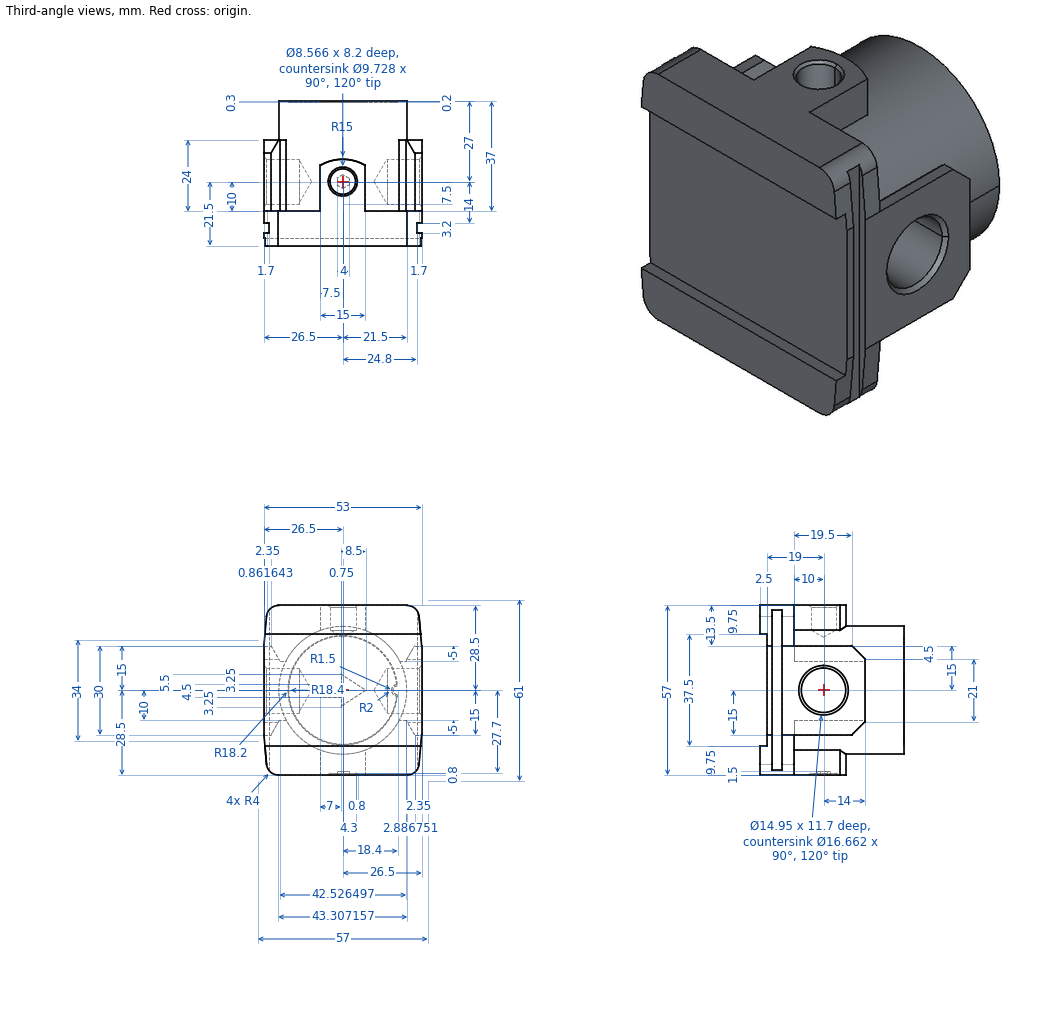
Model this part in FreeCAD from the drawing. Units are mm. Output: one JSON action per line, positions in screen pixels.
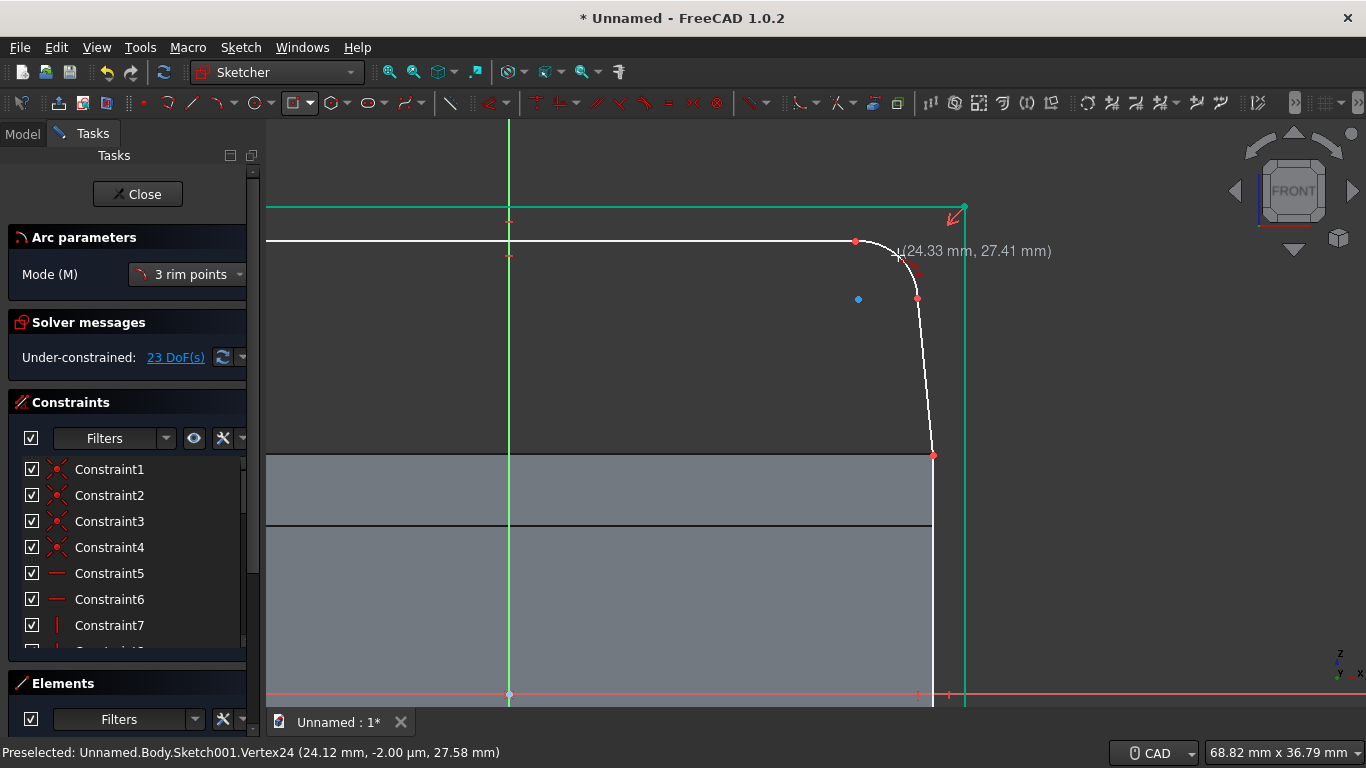
{"action": "scroll", "coordinate": [886, 249], "scroll_direction": "down", "scroll_amount": 5}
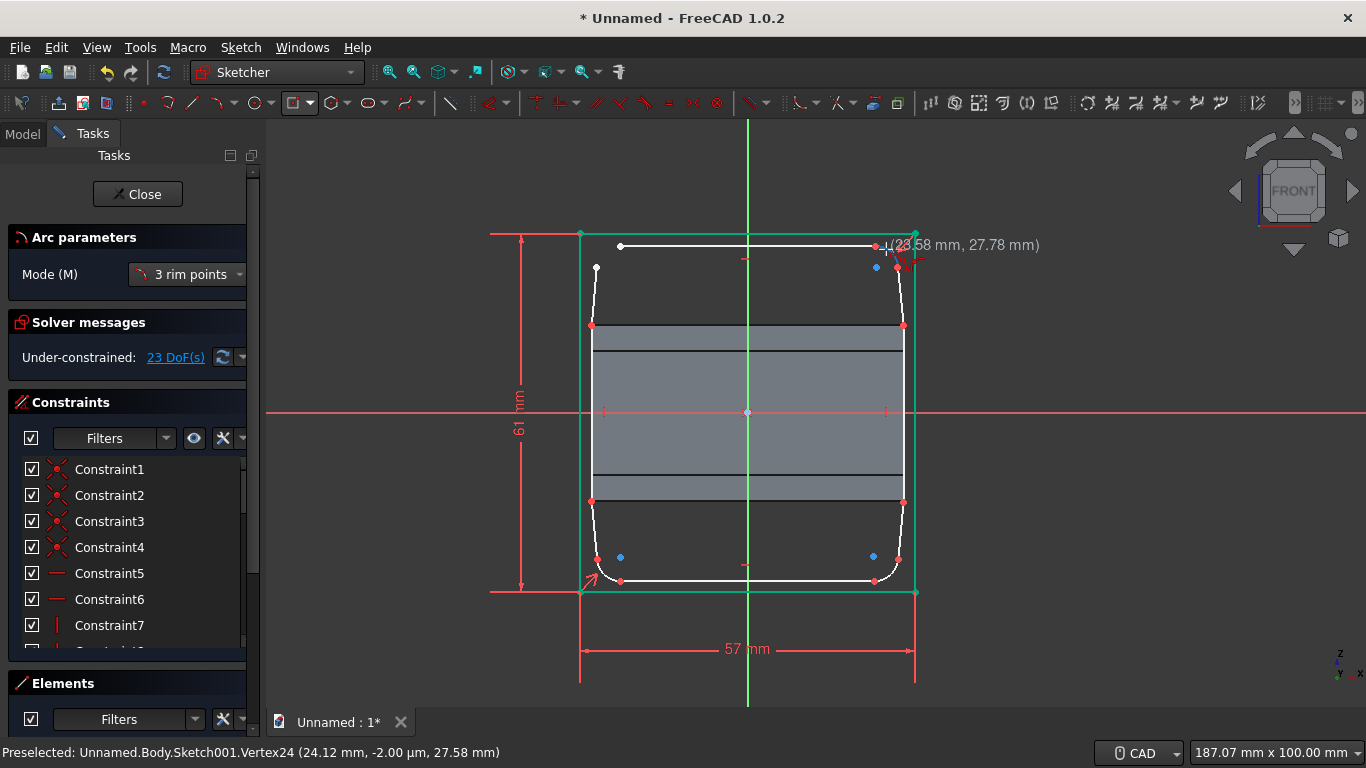
{"action": "scroll", "coordinate": [620, 245], "scroll_direction": "up", "scroll_amount": 2}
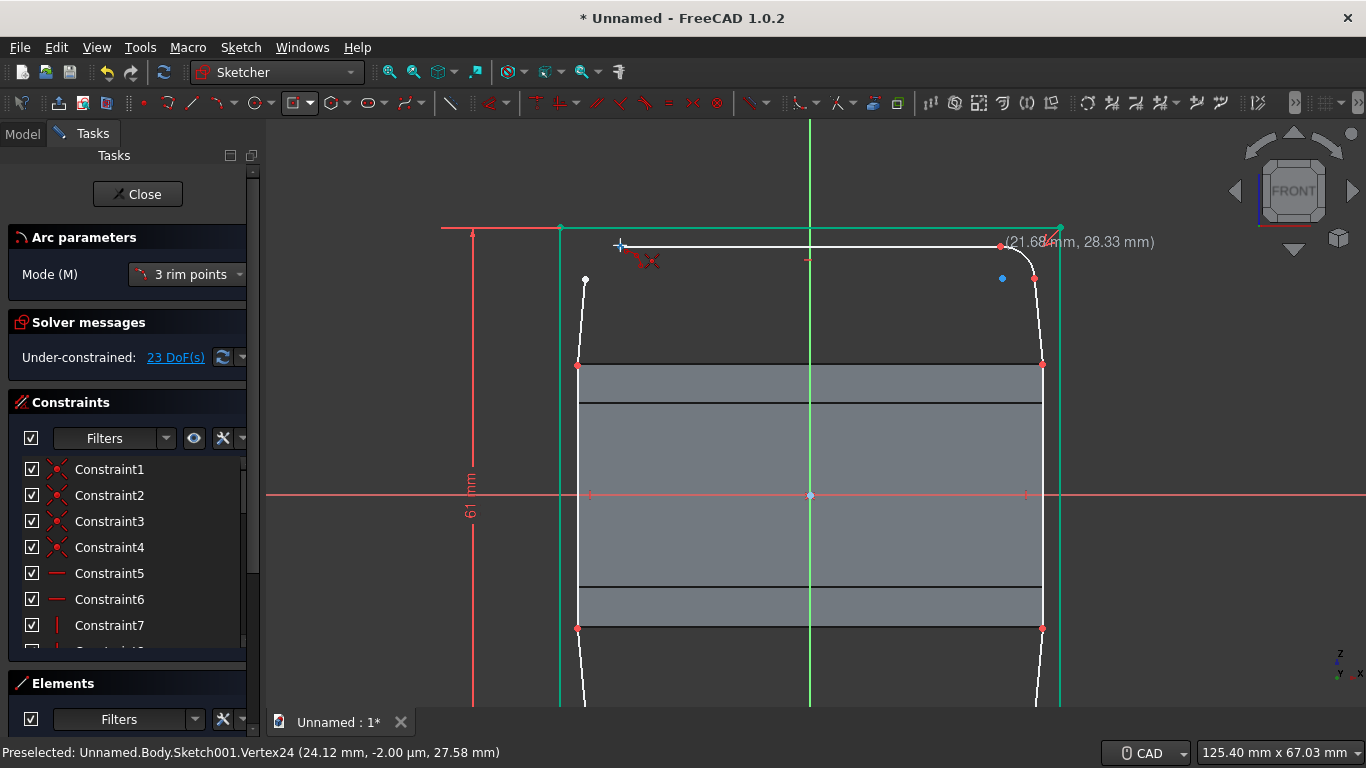
{"action": "left_click", "coordinate": [621, 247]}
{"action": "left_click", "coordinate": [585, 279]}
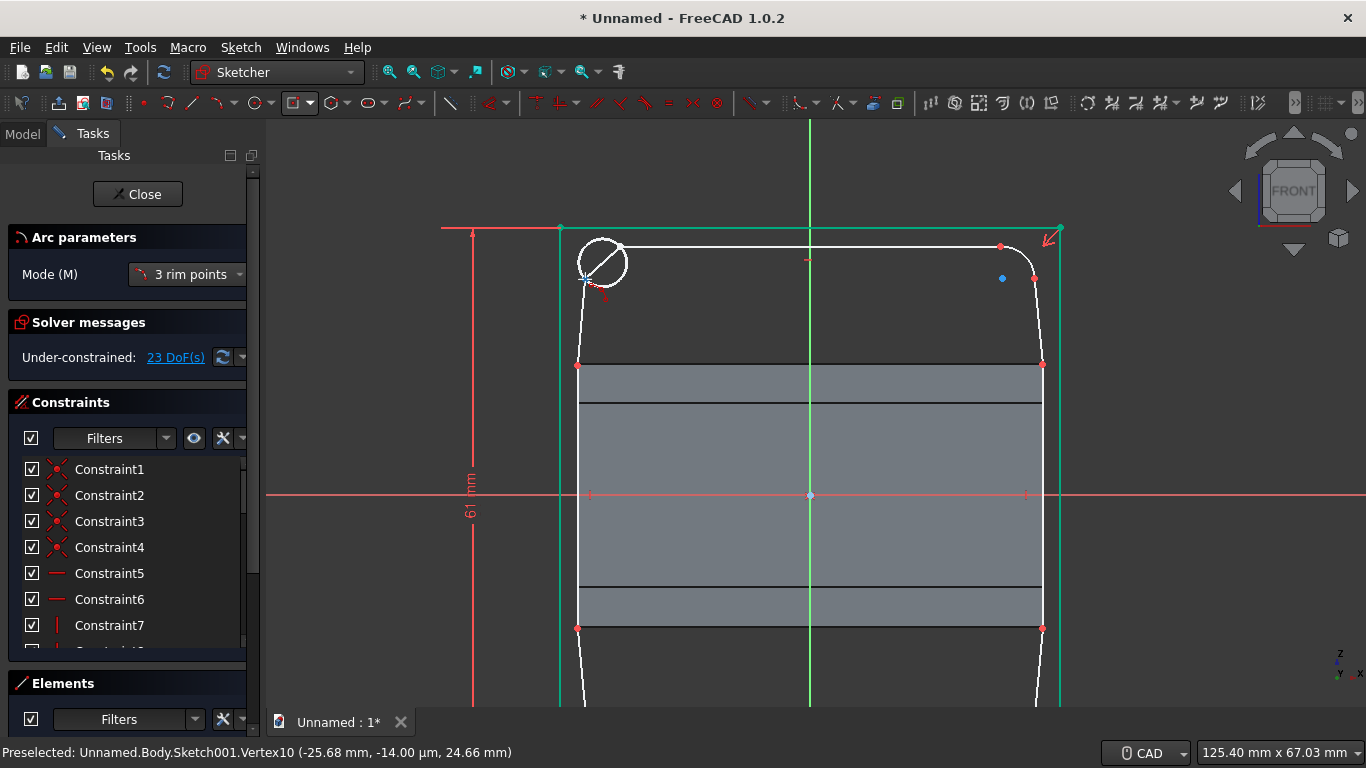
{"action": "scroll", "coordinate": [597, 255], "scroll_direction": "up", "scroll_amount": 3}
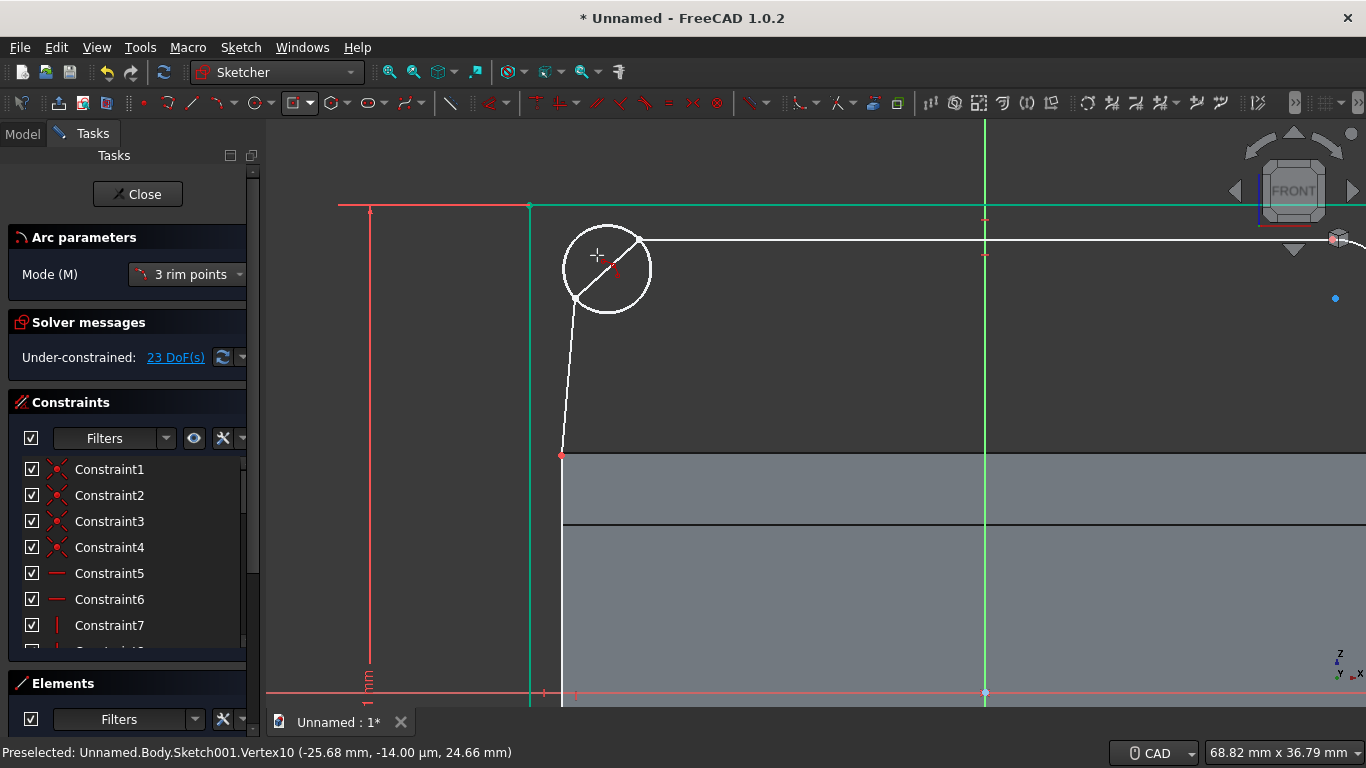
{"action": "left_click", "coordinate": [596, 254]}
{"action": "key", "text": "Escape"}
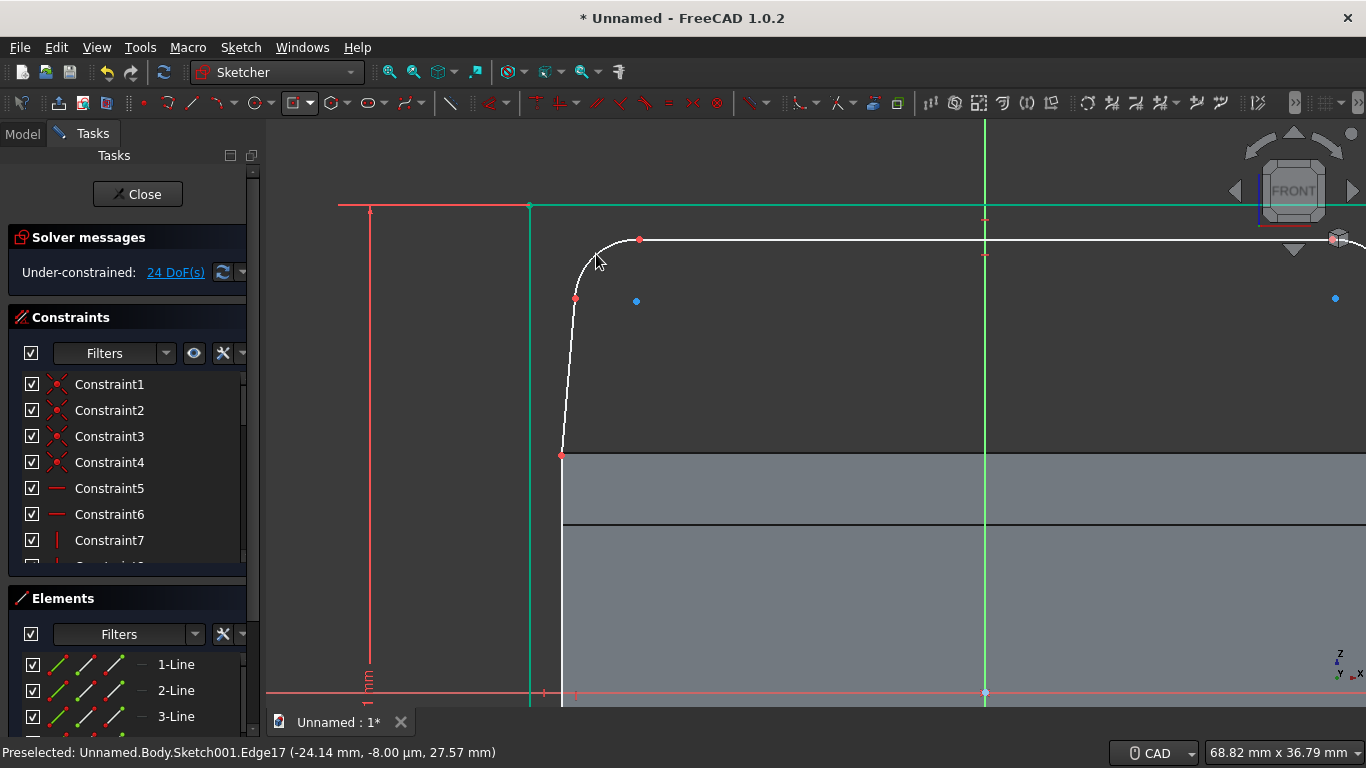
{"action": "left_click", "coordinate": [571, 346]}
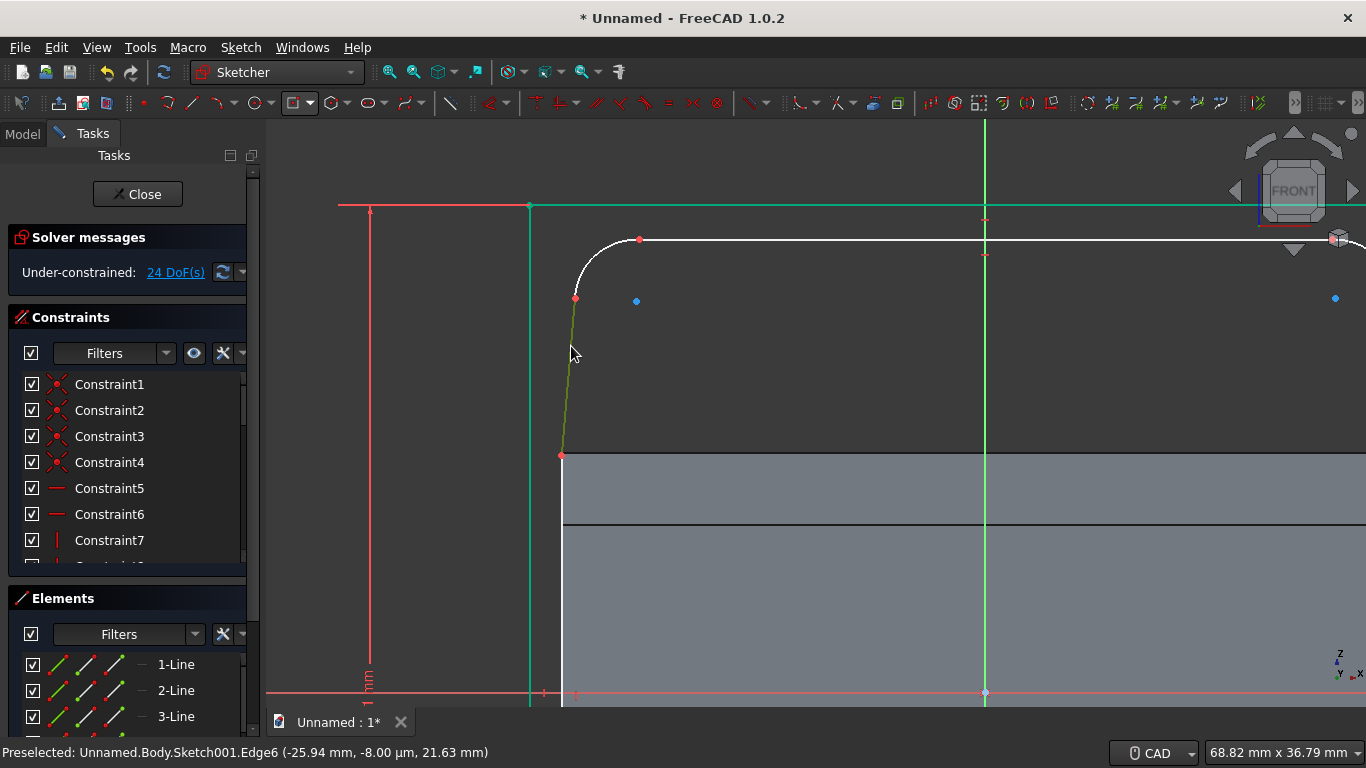
{"action": "left_click", "coordinate": [611, 245]}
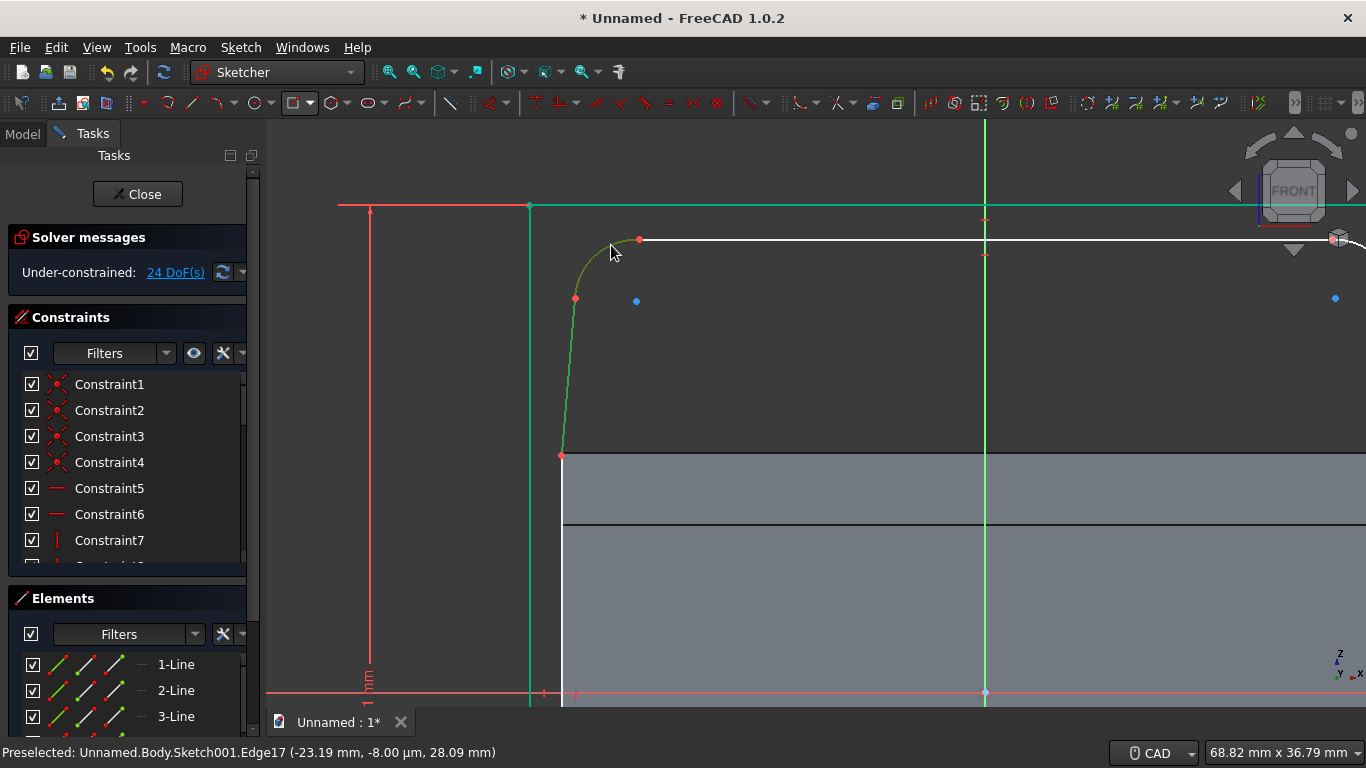
{"action": "left_click", "coordinate": [646, 104]}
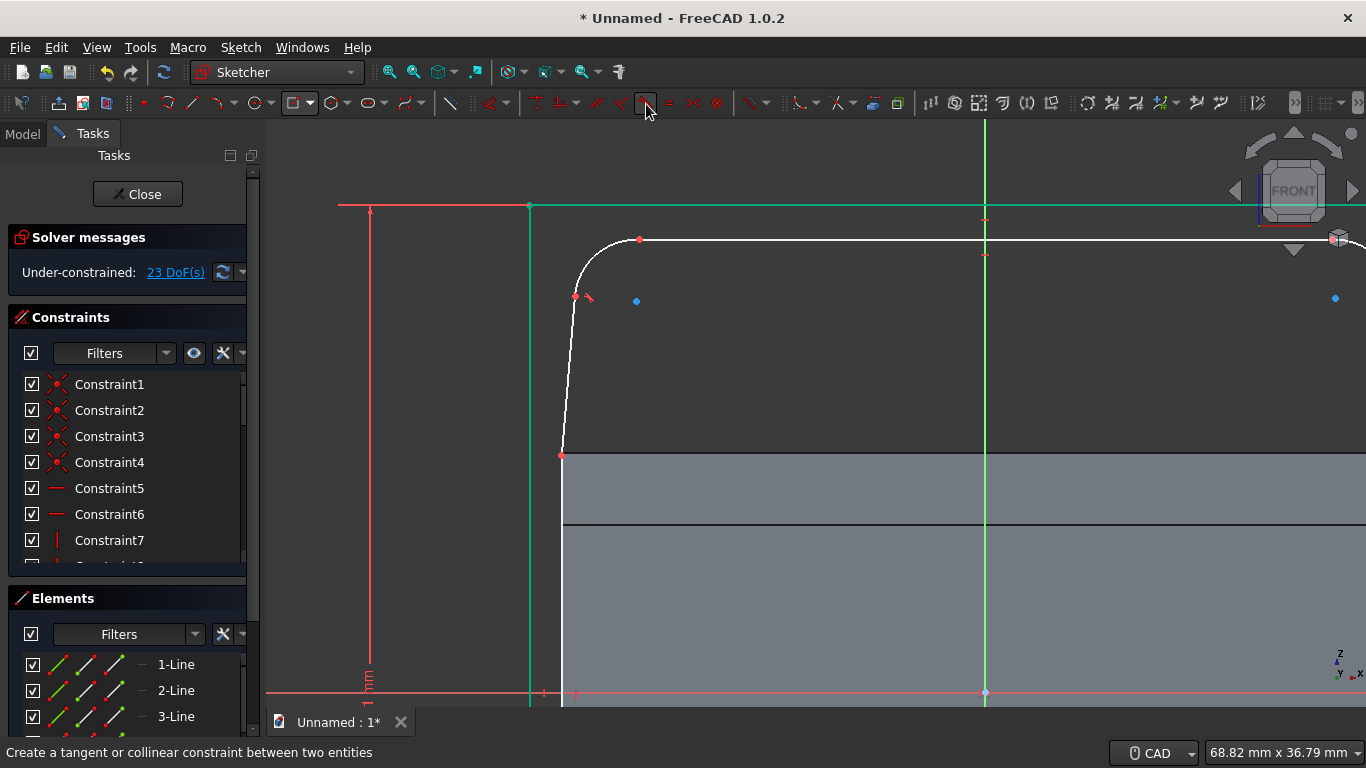
{"action": "scroll", "coordinate": [609, 250], "scroll_direction": "down", "scroll_amount": 5}